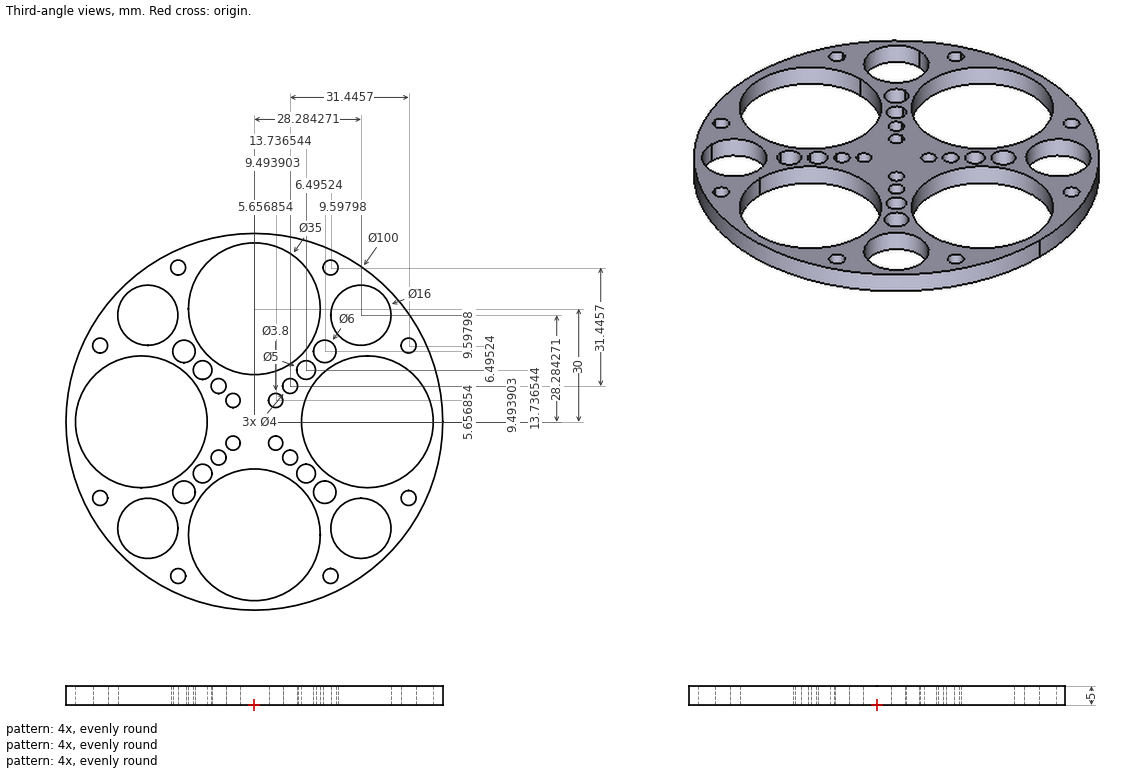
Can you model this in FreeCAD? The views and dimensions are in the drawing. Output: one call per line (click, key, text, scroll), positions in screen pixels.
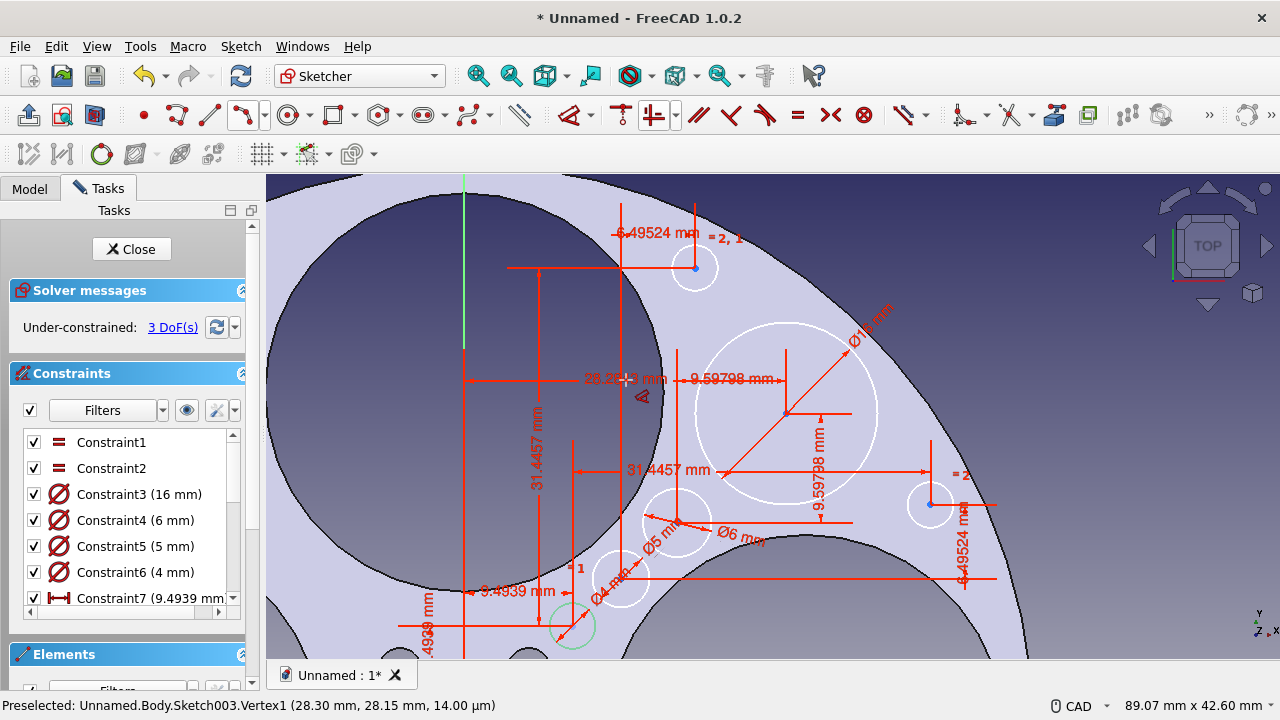
click(786, 414)
click(430, 522)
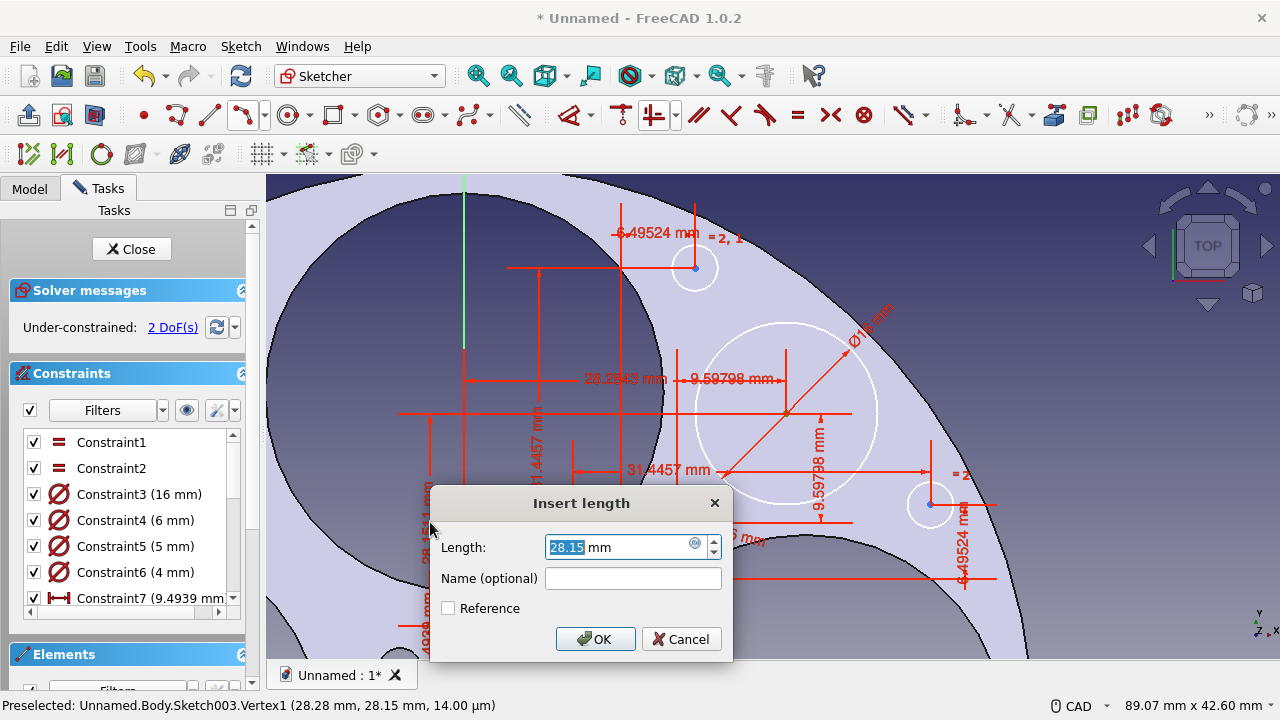
text(28.284271)
key(Return)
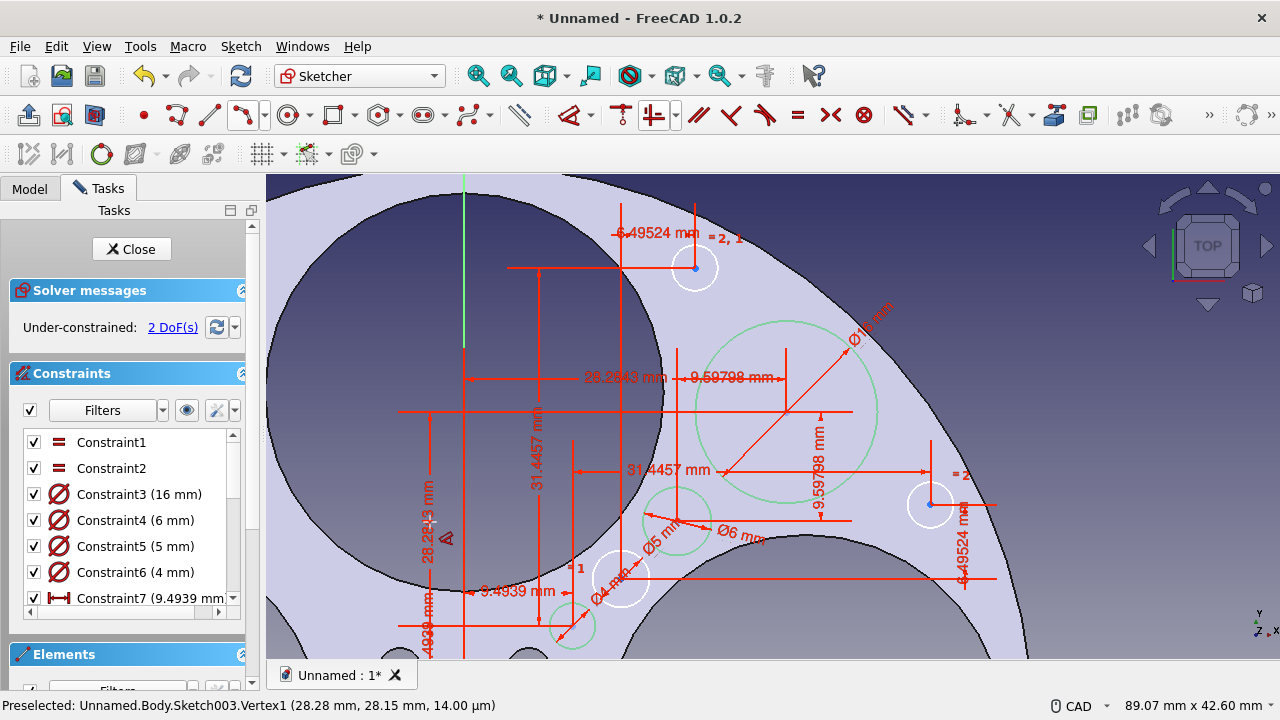
click(621, 579)
click(543, 545)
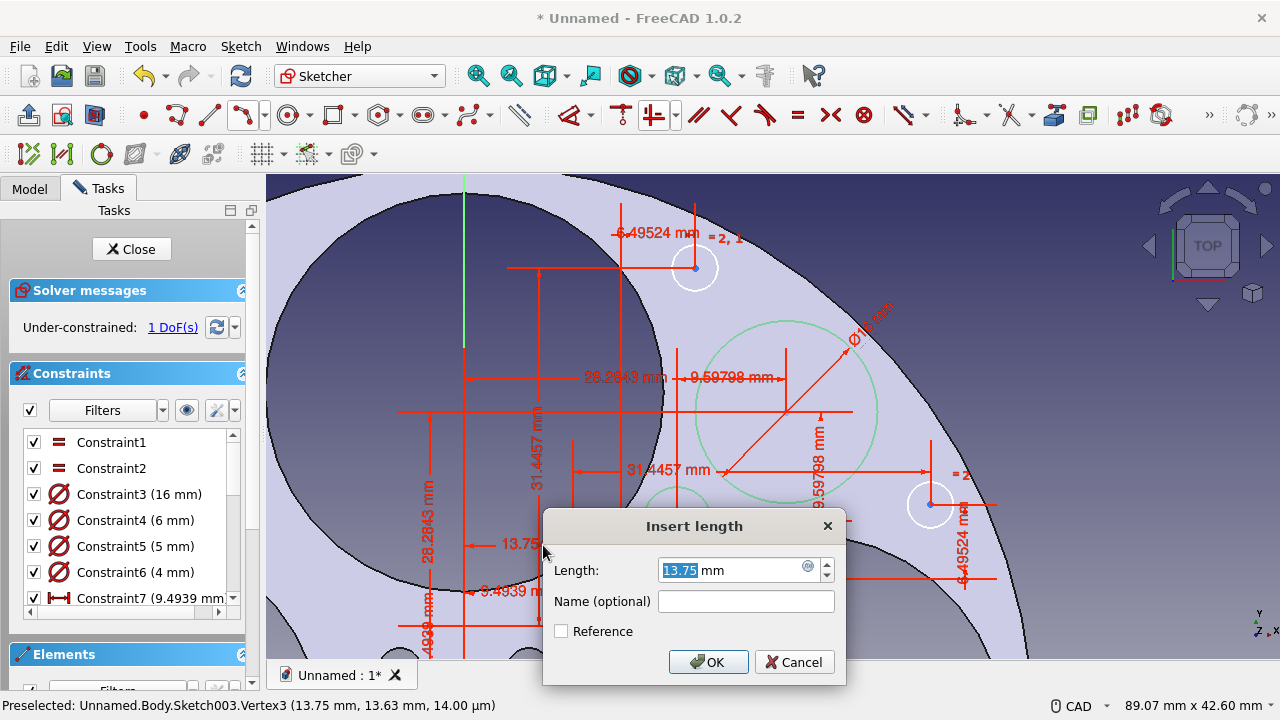
text(13.736544)
key(Return)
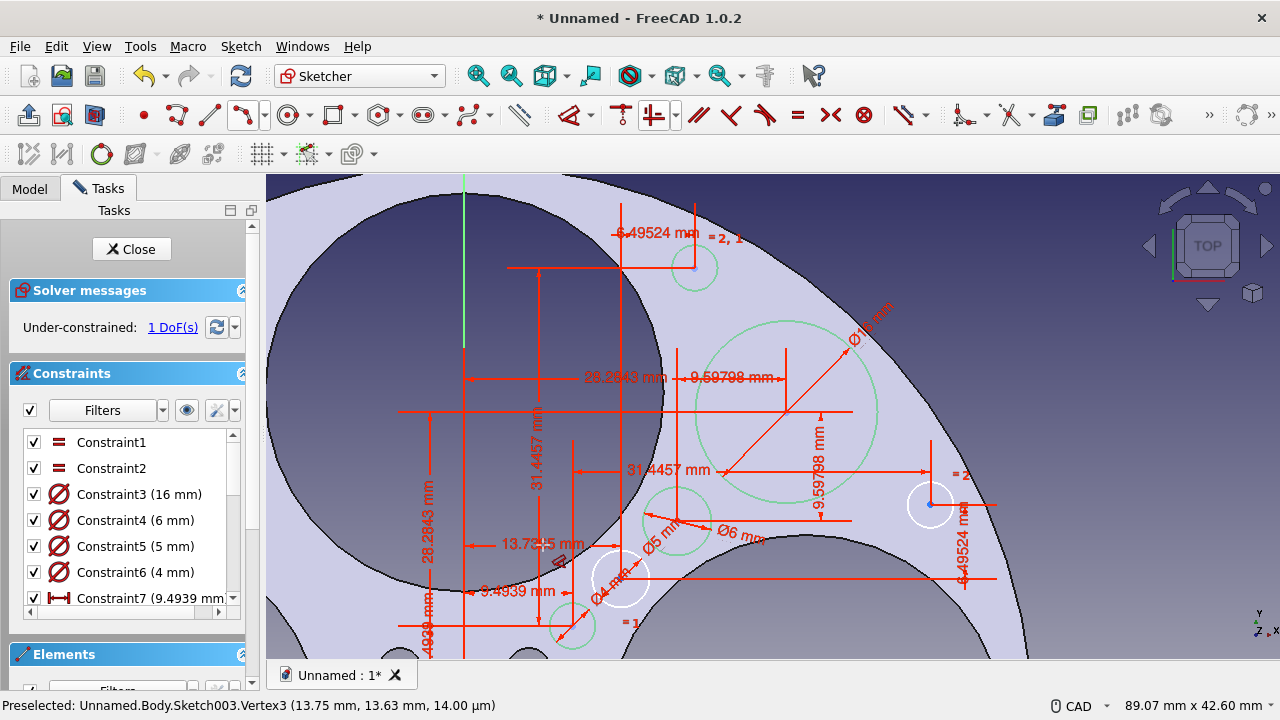
click(621, 579)
click(430, 605)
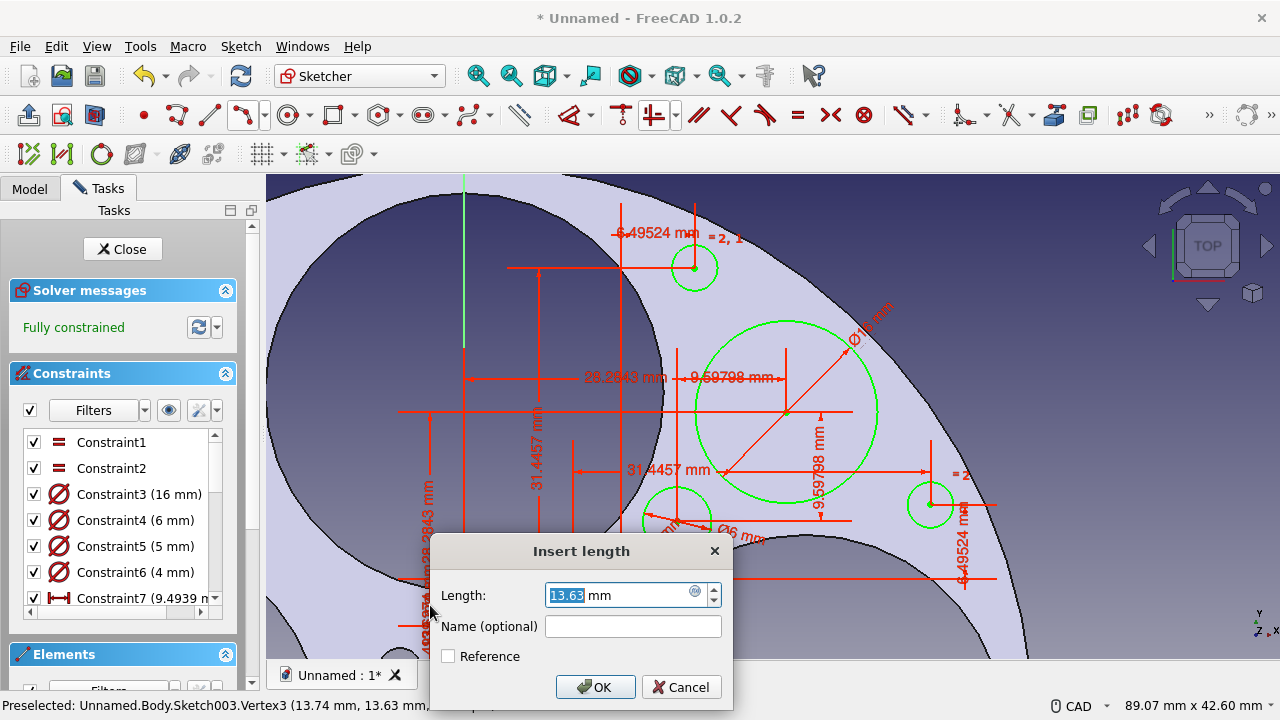
text(13.736544)
key(Return)
key(Escape)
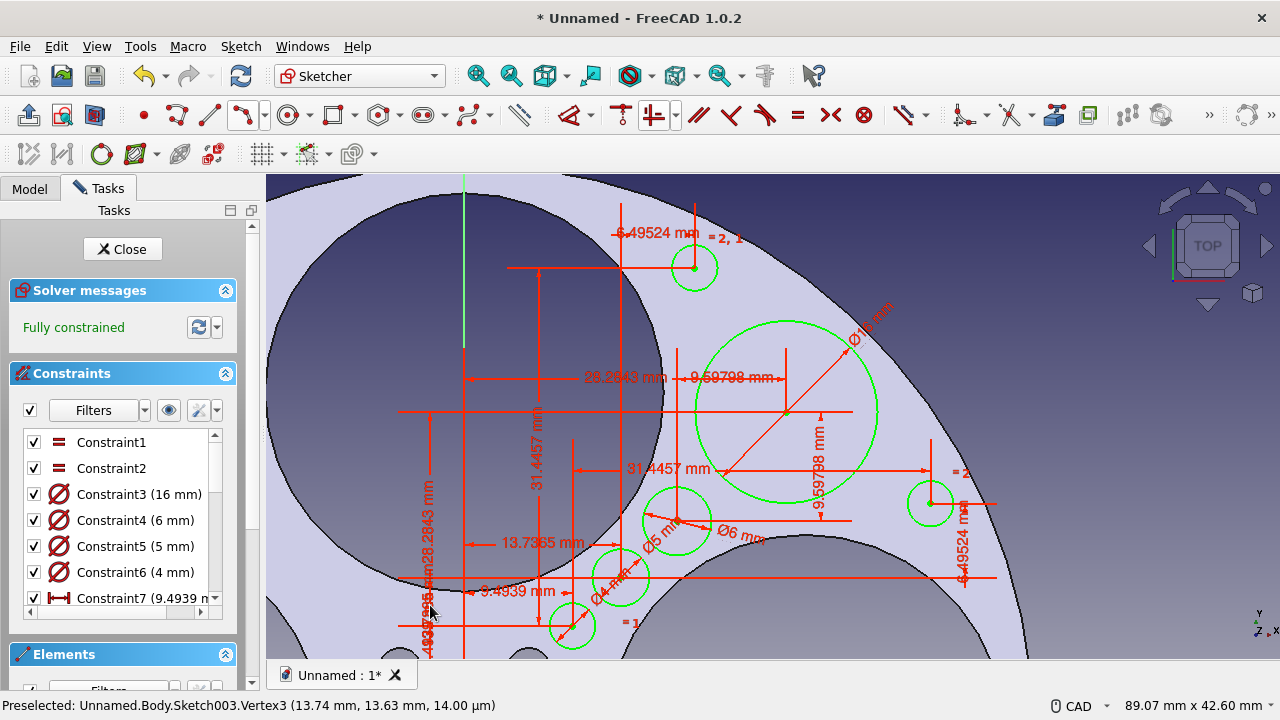
click(123, 249)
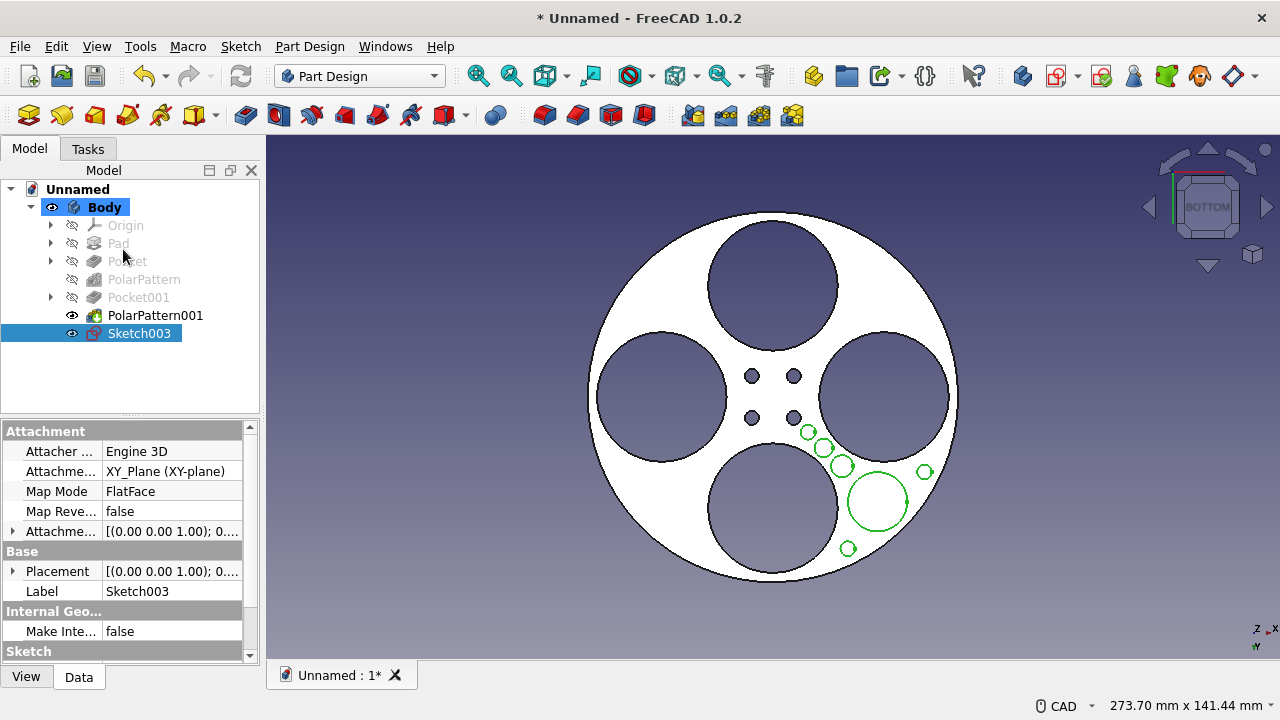
click(246, 116)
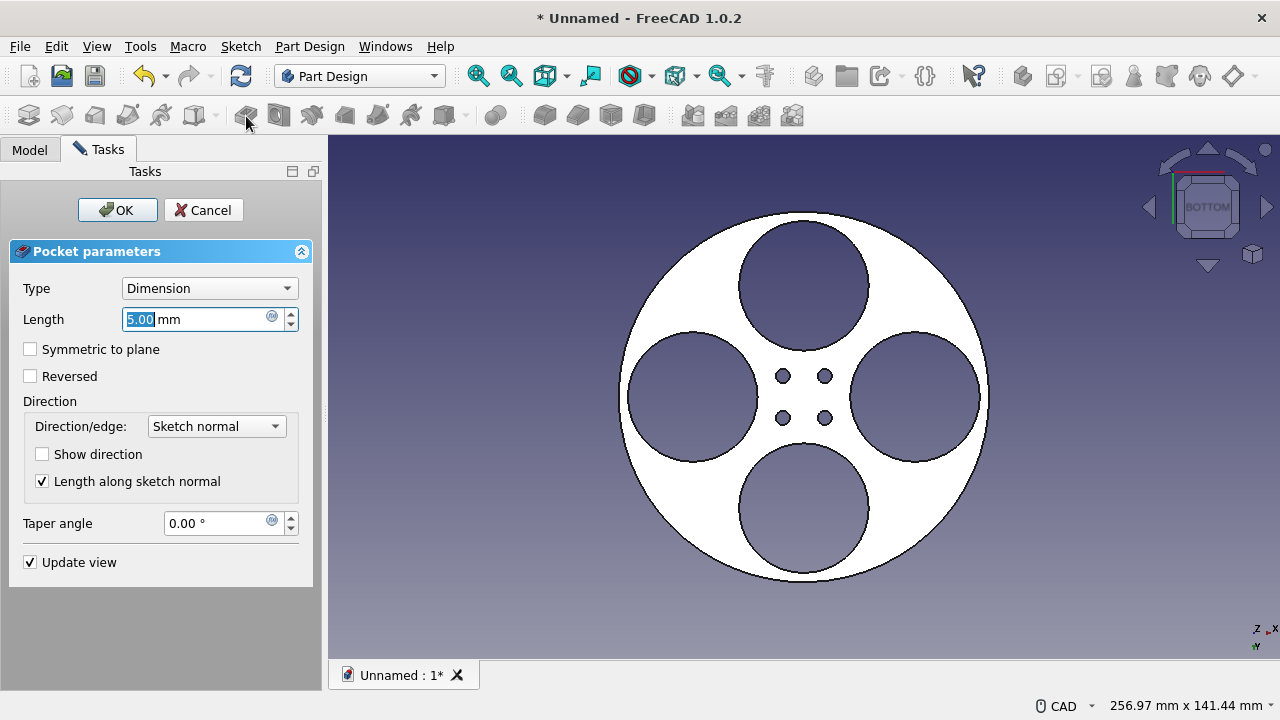
click(210, 288)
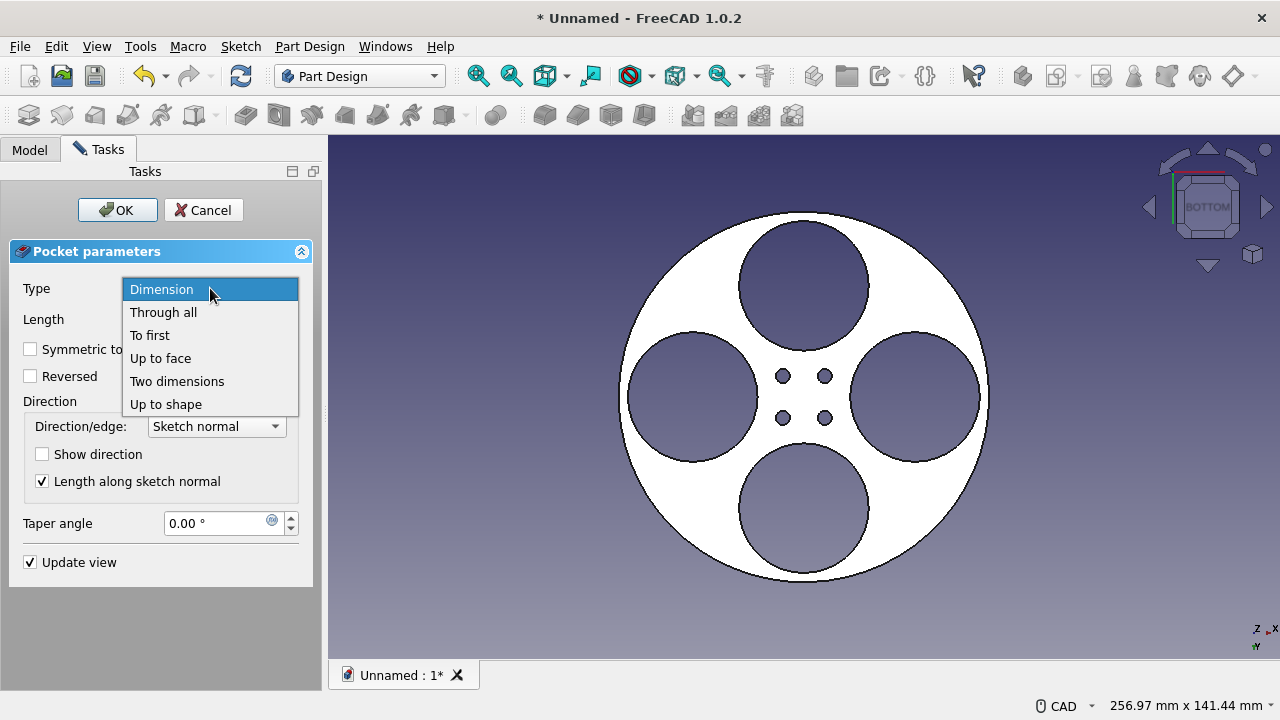
click(208, 312)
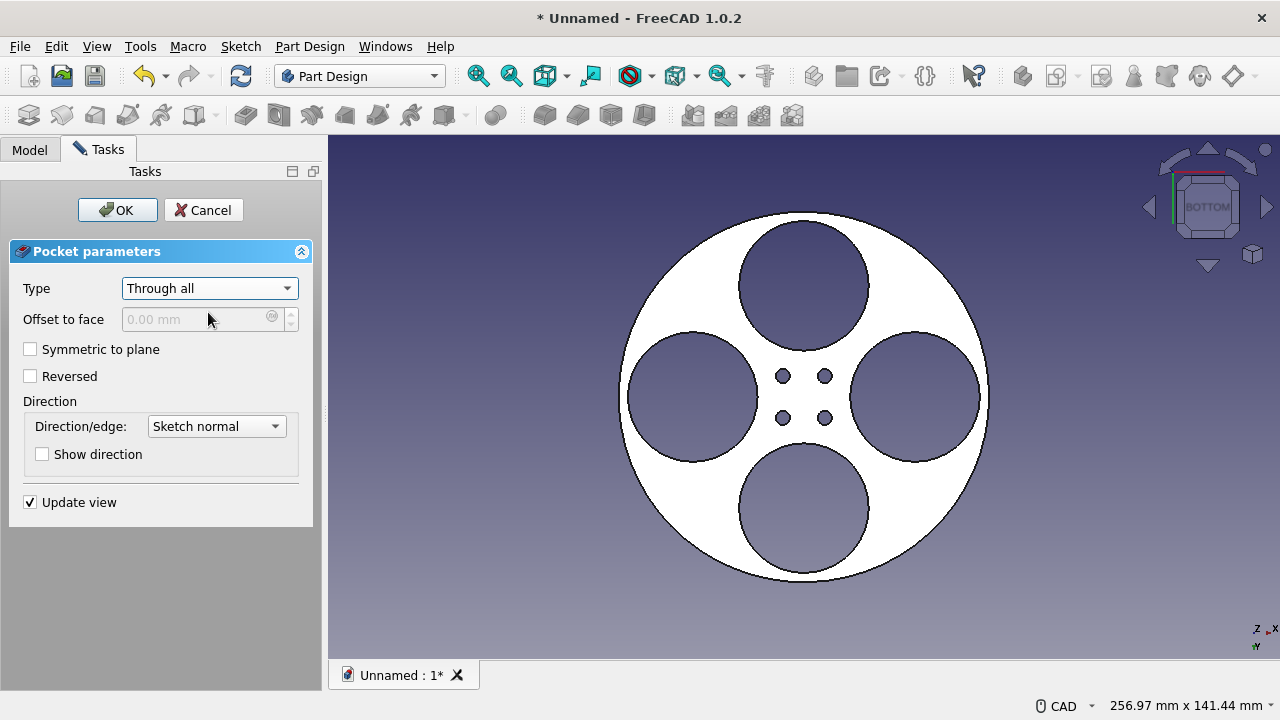
click(31, 376)